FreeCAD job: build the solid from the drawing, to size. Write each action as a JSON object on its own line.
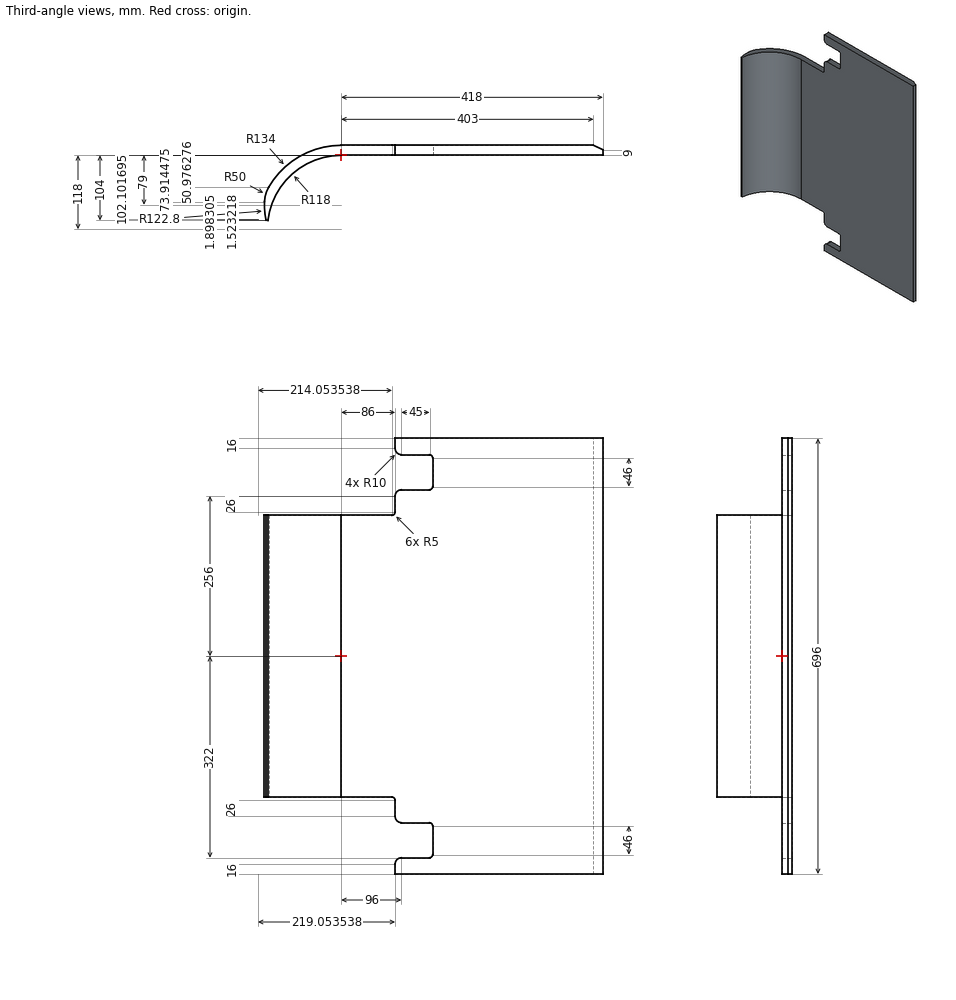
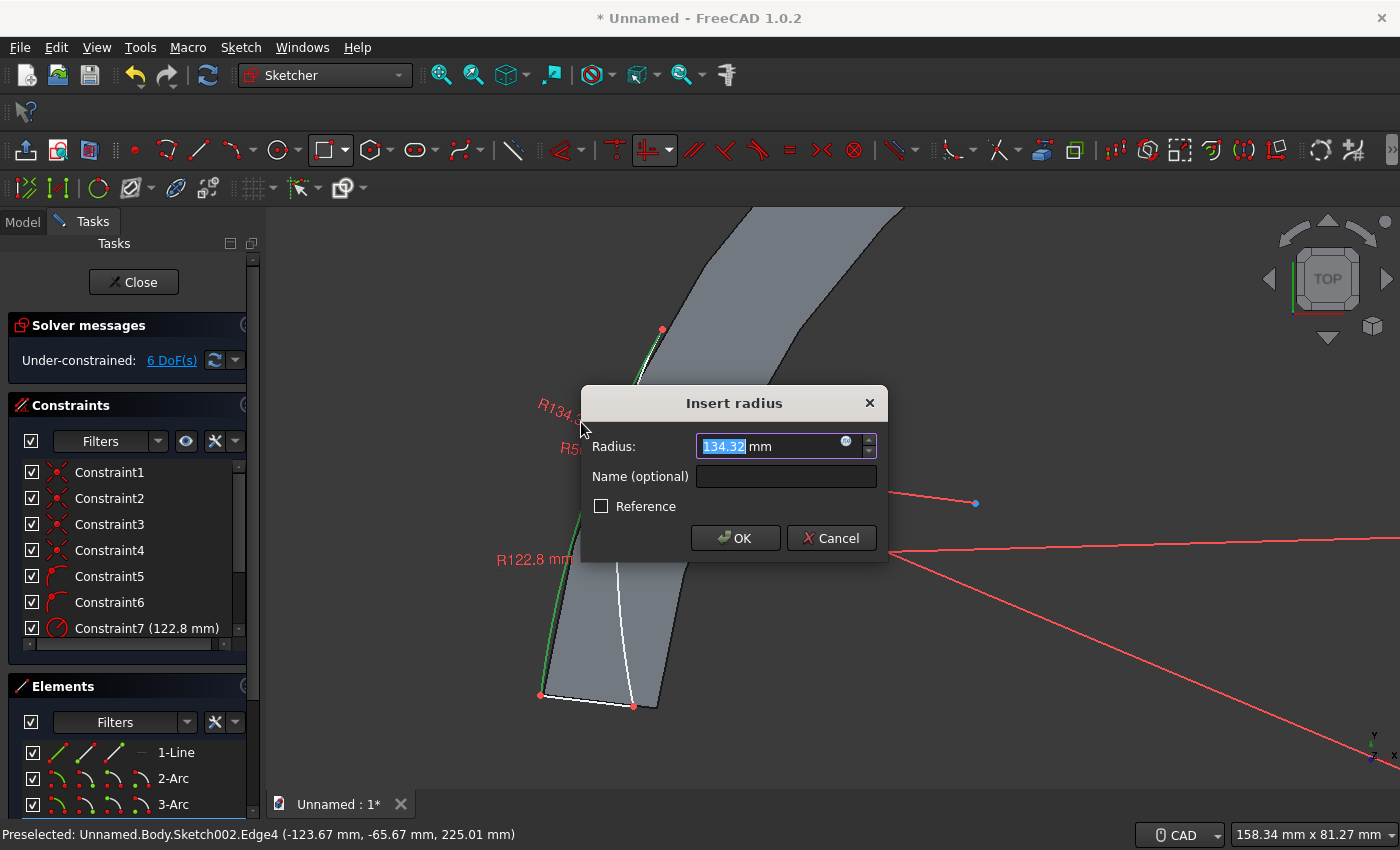
{"action": "type", "text": "134"}
{"action": "key", "text": "Return"}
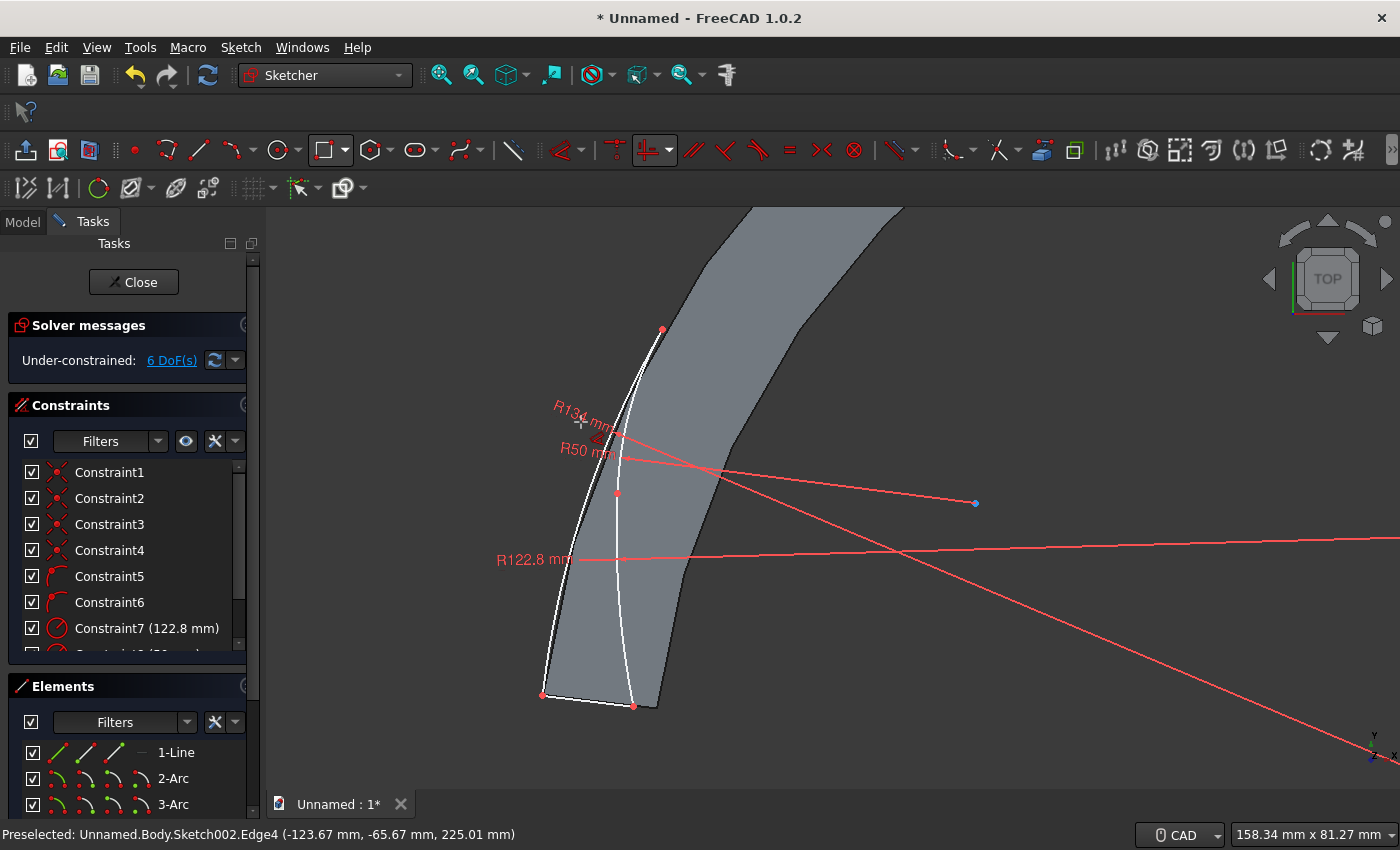
{"action": "scroll", "coordinate": [294, 459], "scroll_direction": "down", "scroll_amount": 2}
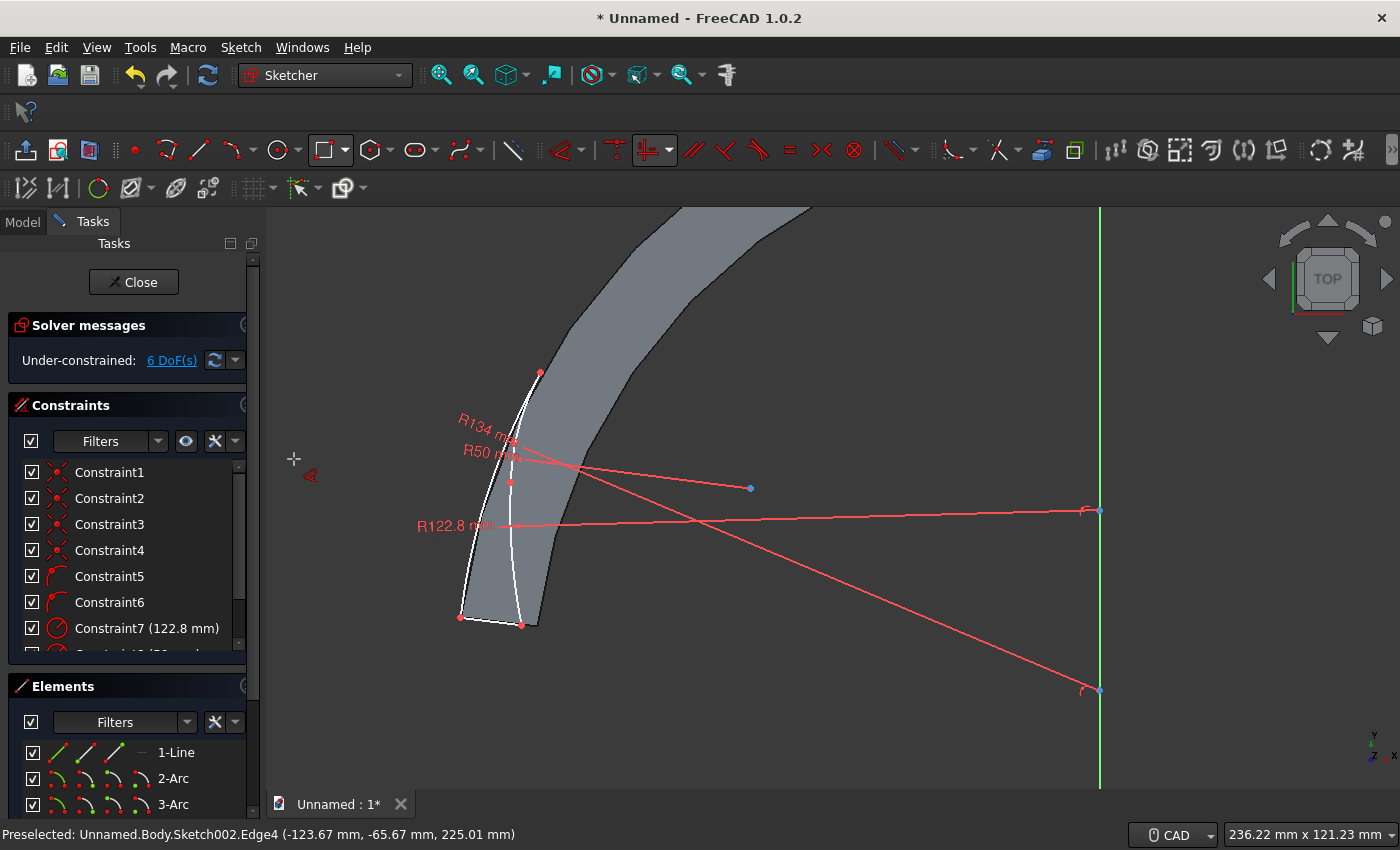
{"action": "left_click", "coordinate": [1100, 510]}
{"action": "left_click", "coordinate": [1134, 373]}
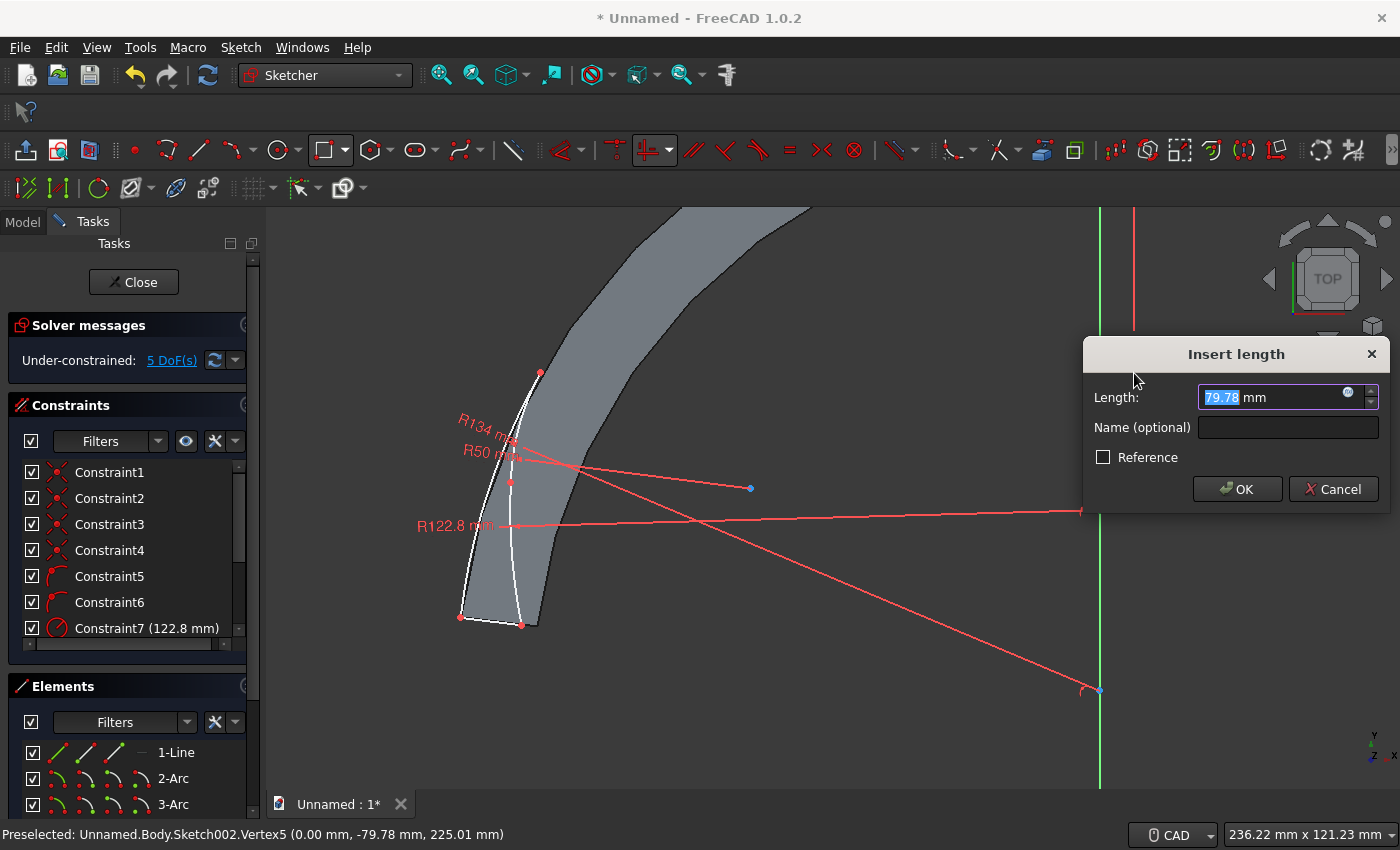
{"action": "type", "text": "79"}
{"action": "key", "text": "Return"}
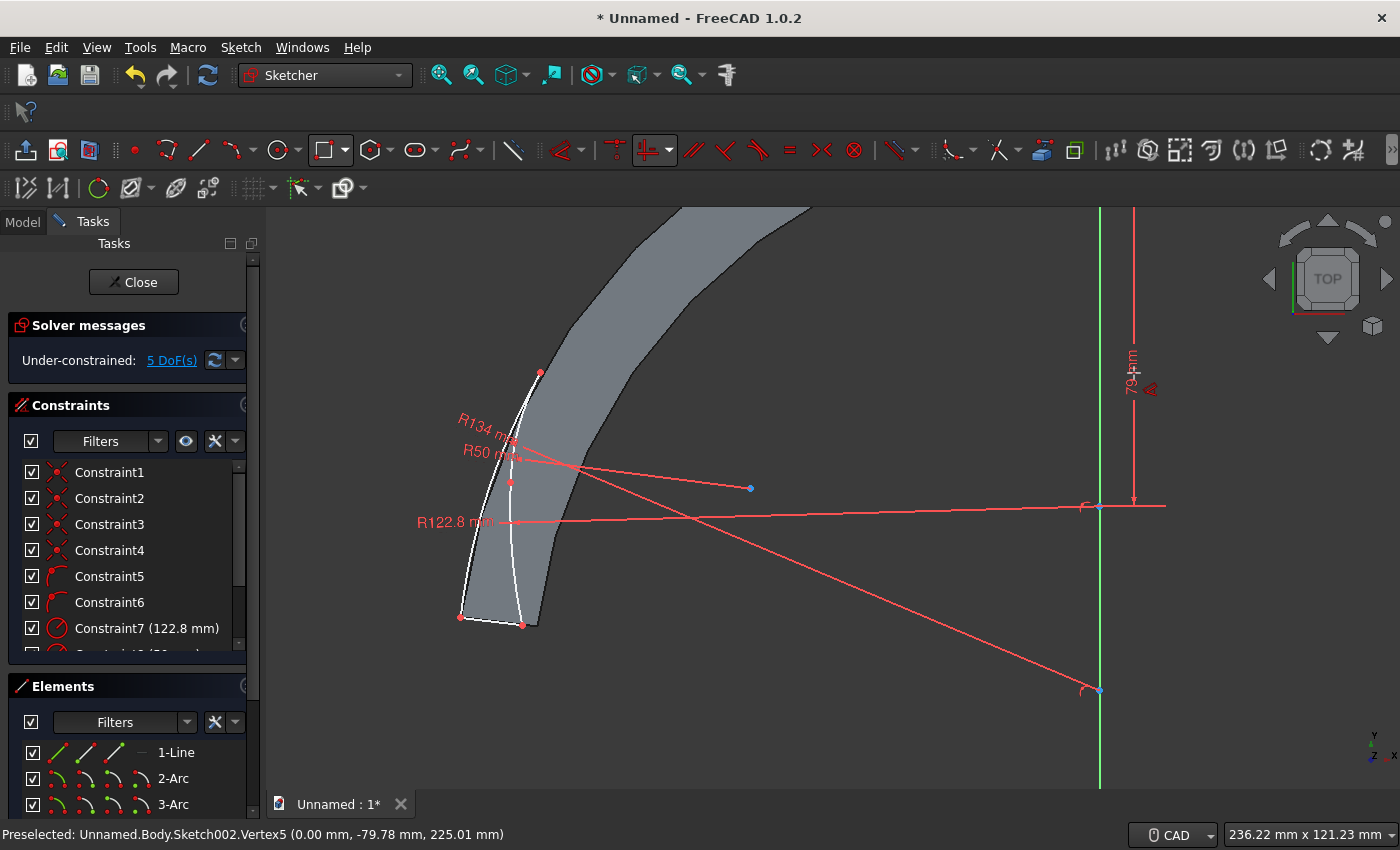
{"action": "left_click", "coordinate": [1100, 691]}
{"action": "left_click", "coordinate": [1134, 463]}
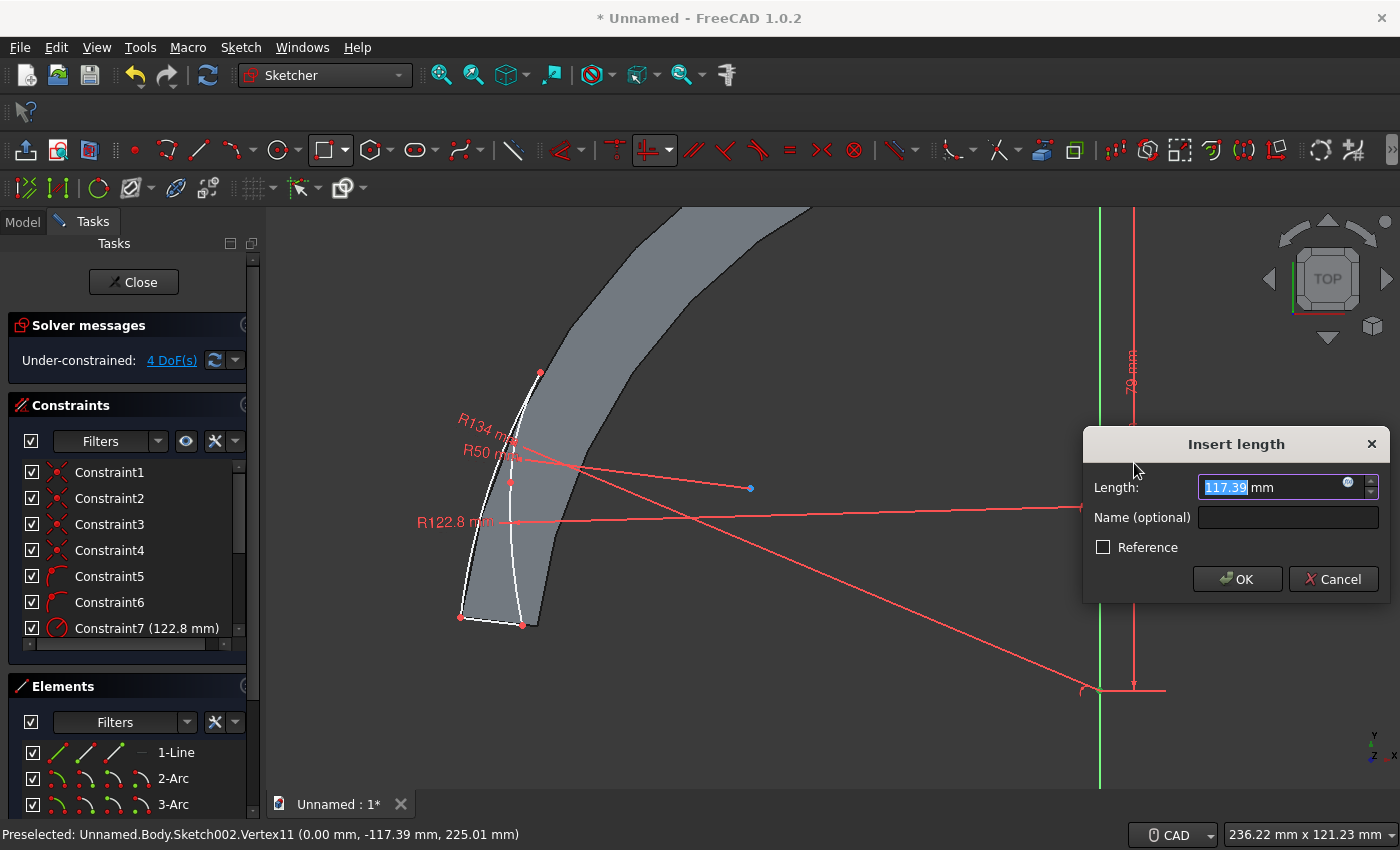
{"action": "type", "text": "118"}
{"action": "key", "text": "Return"}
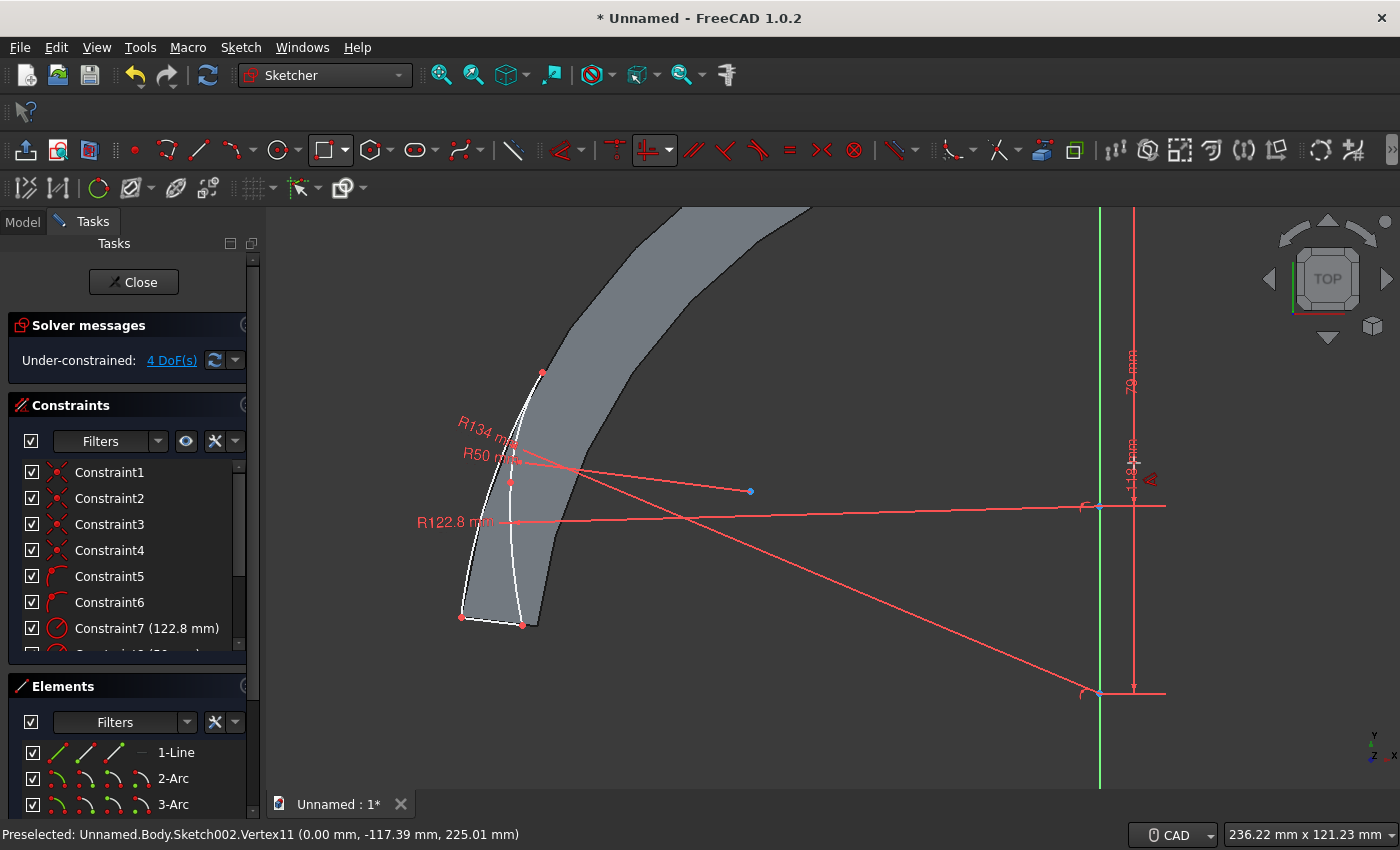
{"action": "scroll", "coordinate": [479, 620], "scroll_direction": "up", "scroll_amount": 9}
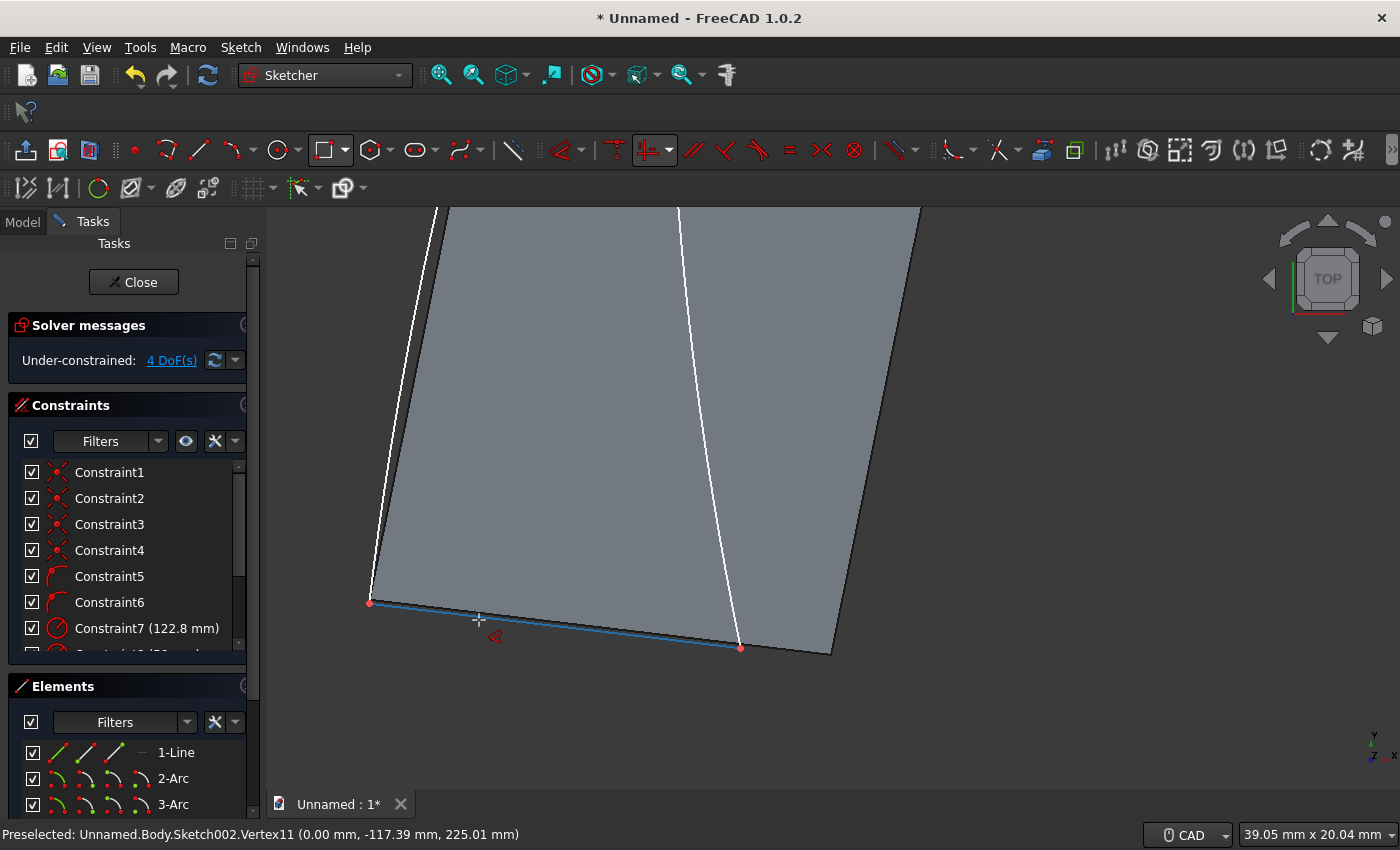
{"action": "left_click", "coordinate": [481, 617]}
{"action": "left_click", "coordinate": [335, 626]}